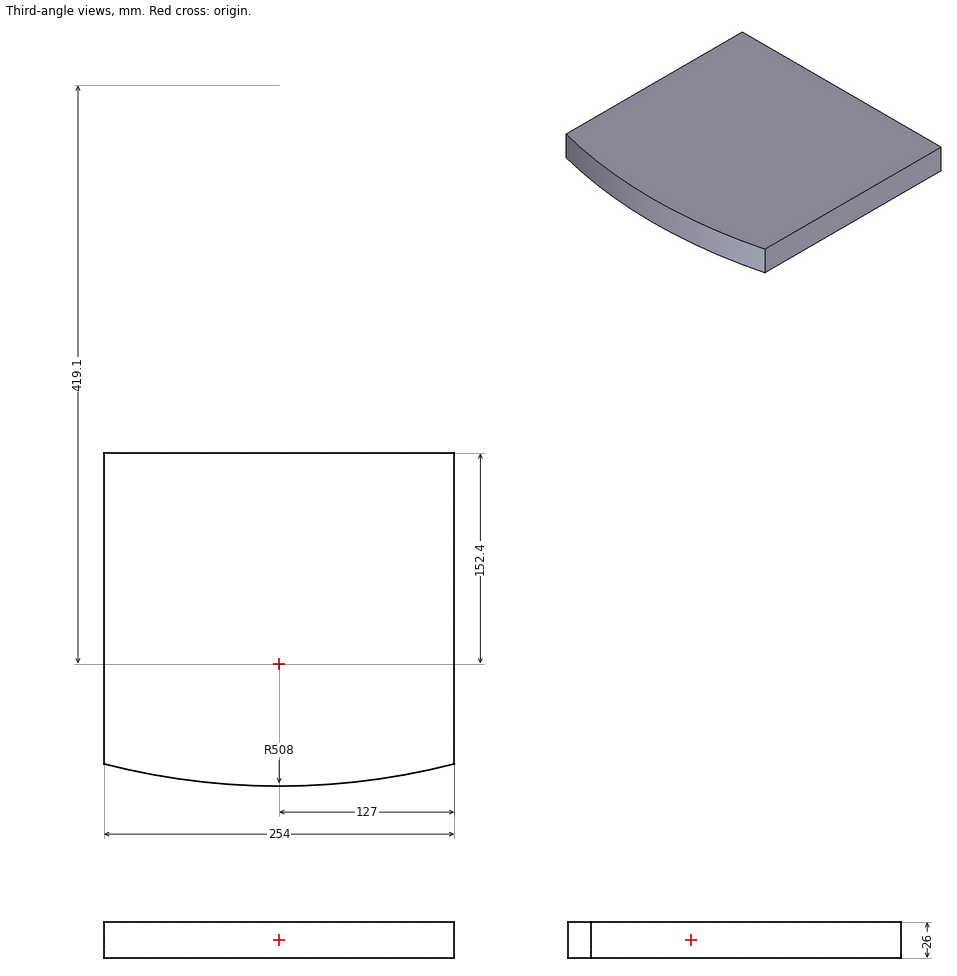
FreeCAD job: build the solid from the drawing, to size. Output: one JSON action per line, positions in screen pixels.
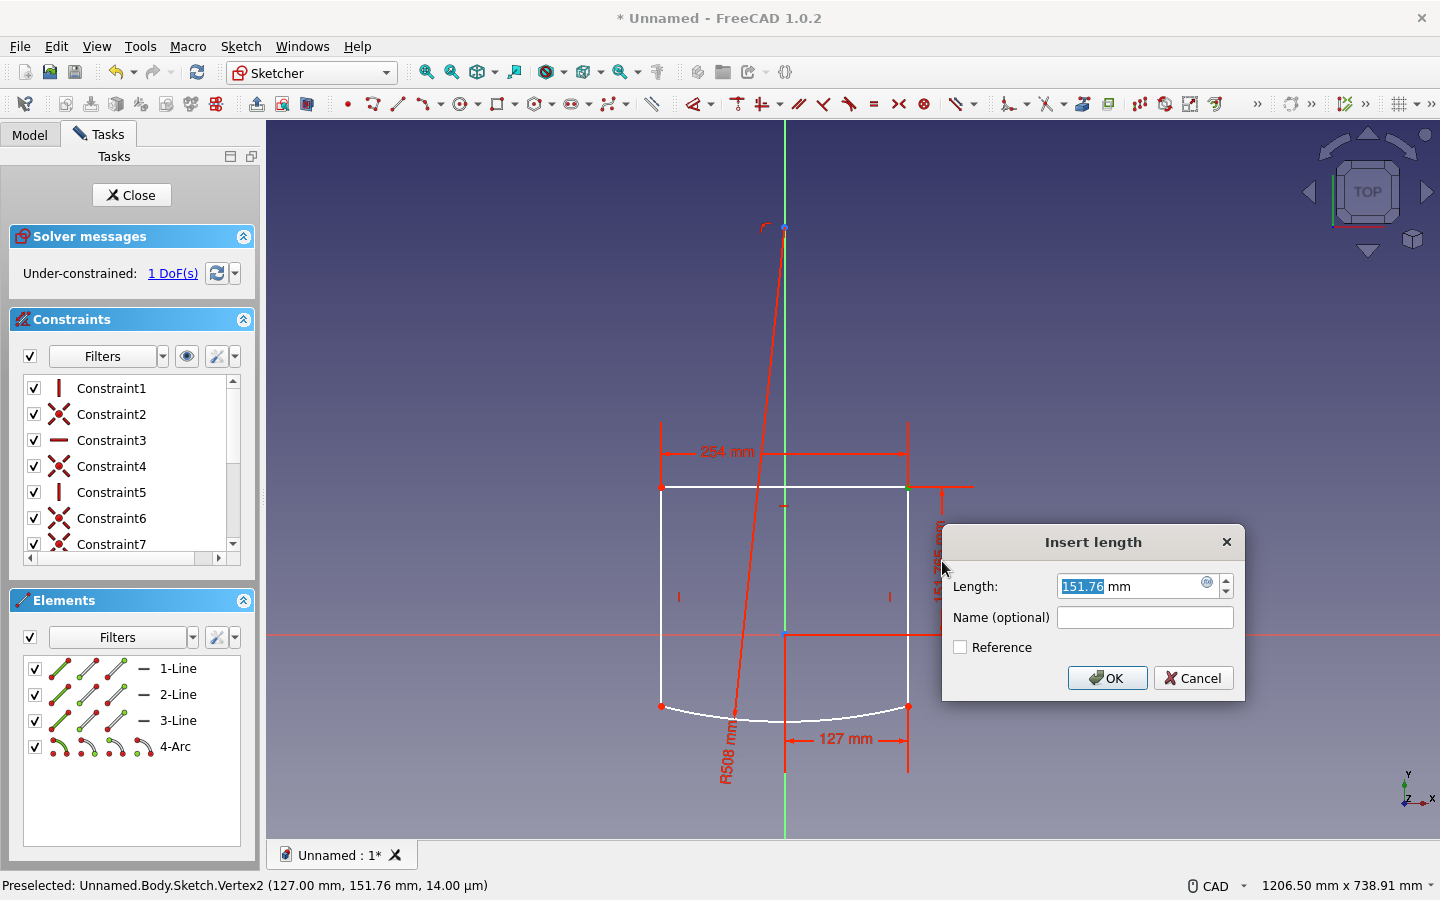
{"action": "type", "text": "152.4"}
{"action": "key", "text": "Return"}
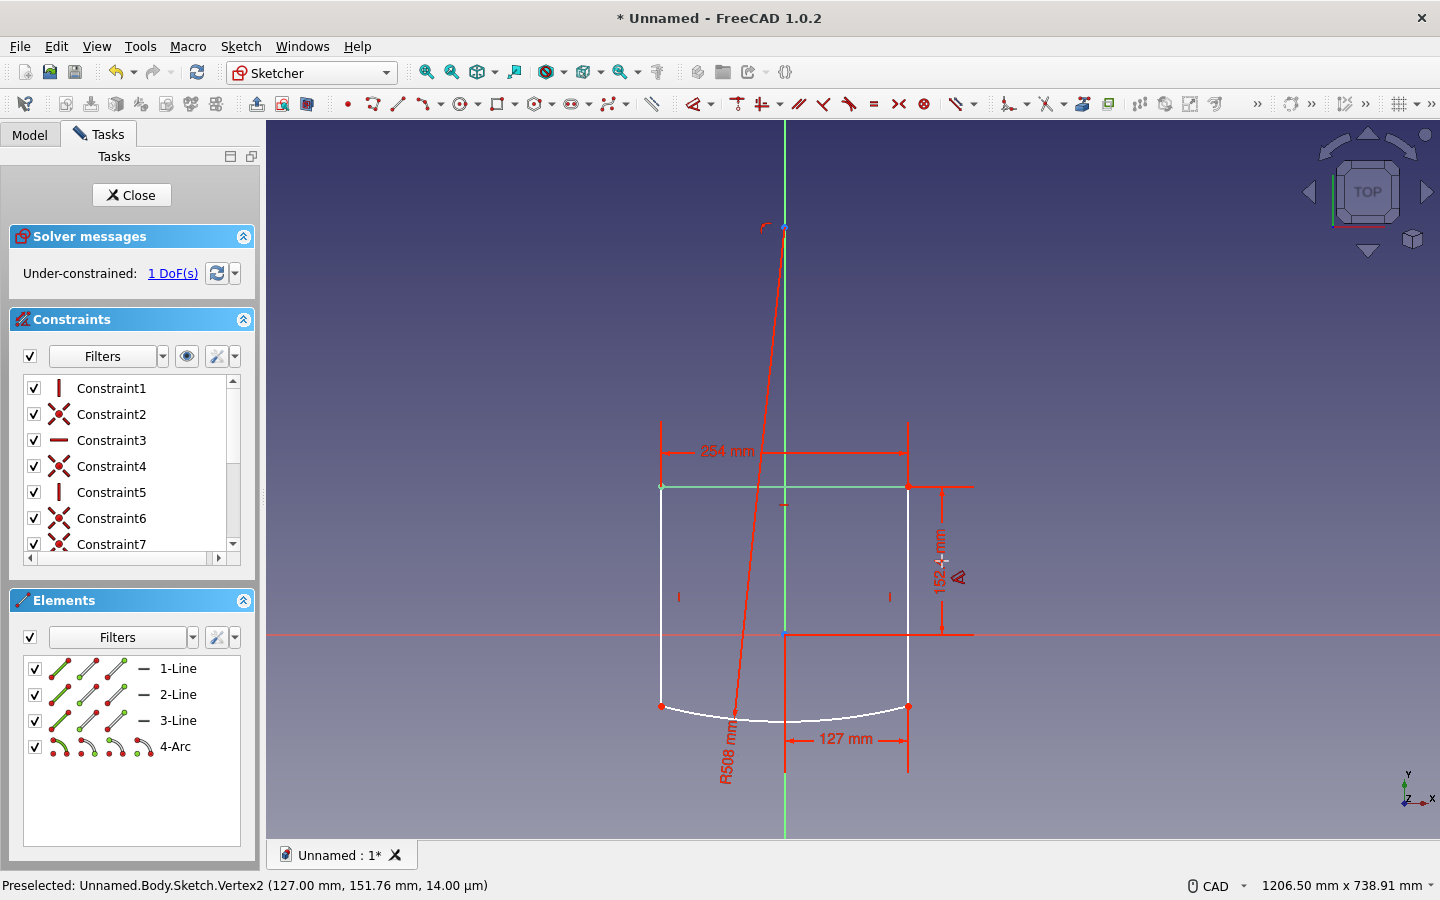
{"action": "left_click", "coordinate": [785, 227]}
{"action": "left_click", "coordinate": [819, 431]}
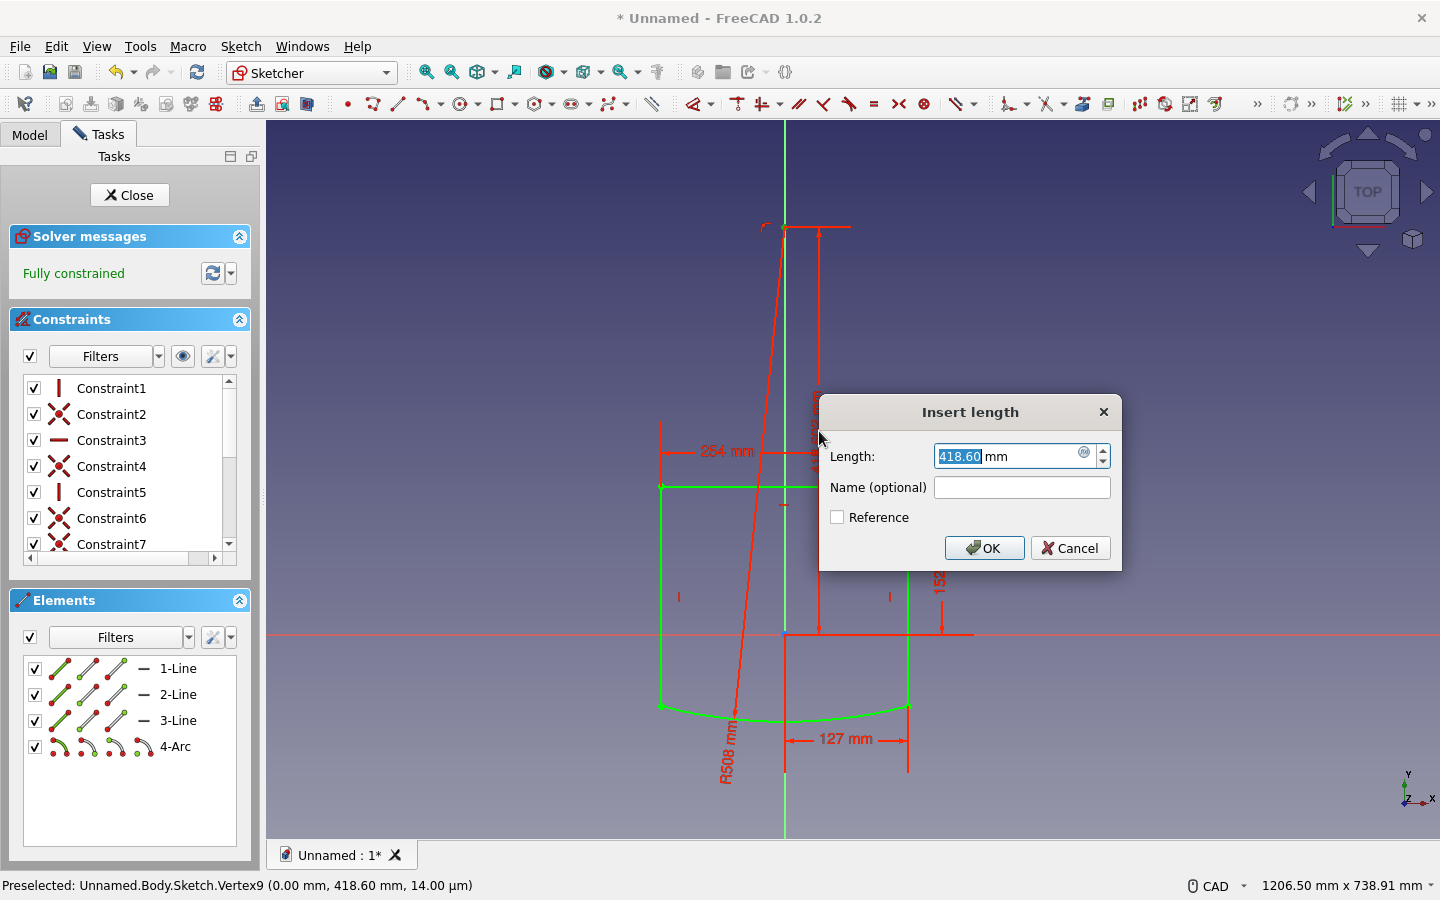
{"action": "type", "text": "419.1"}
{"action": "key", "text": "Return"}
{"action": "key", "text": "Escape"}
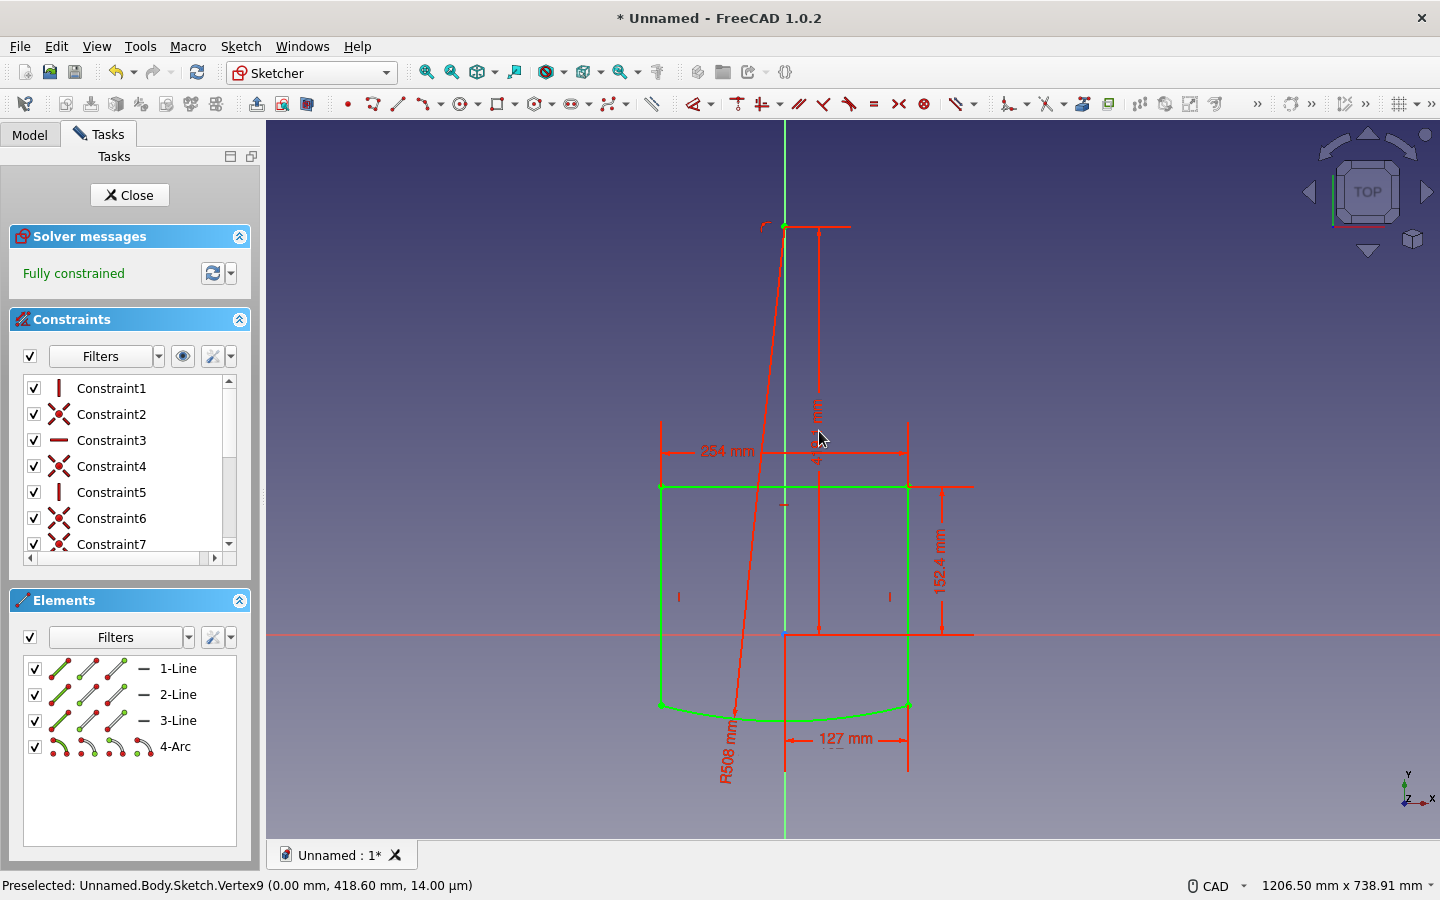
{"action": "left_click", "coordinate": [130, 195]}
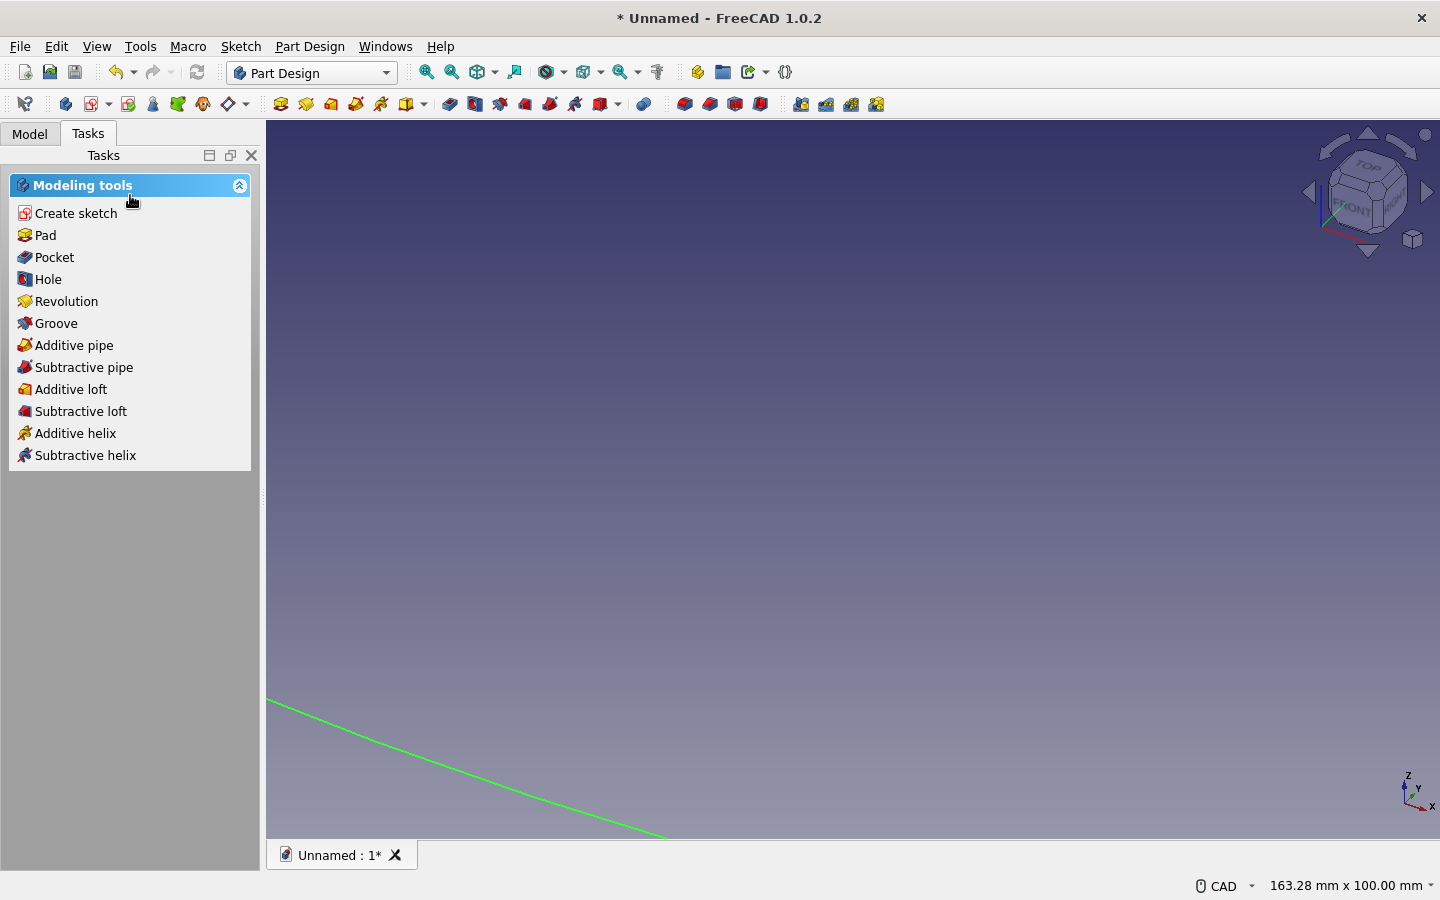
{"action": "left_click", "coordinate": [281, 104]}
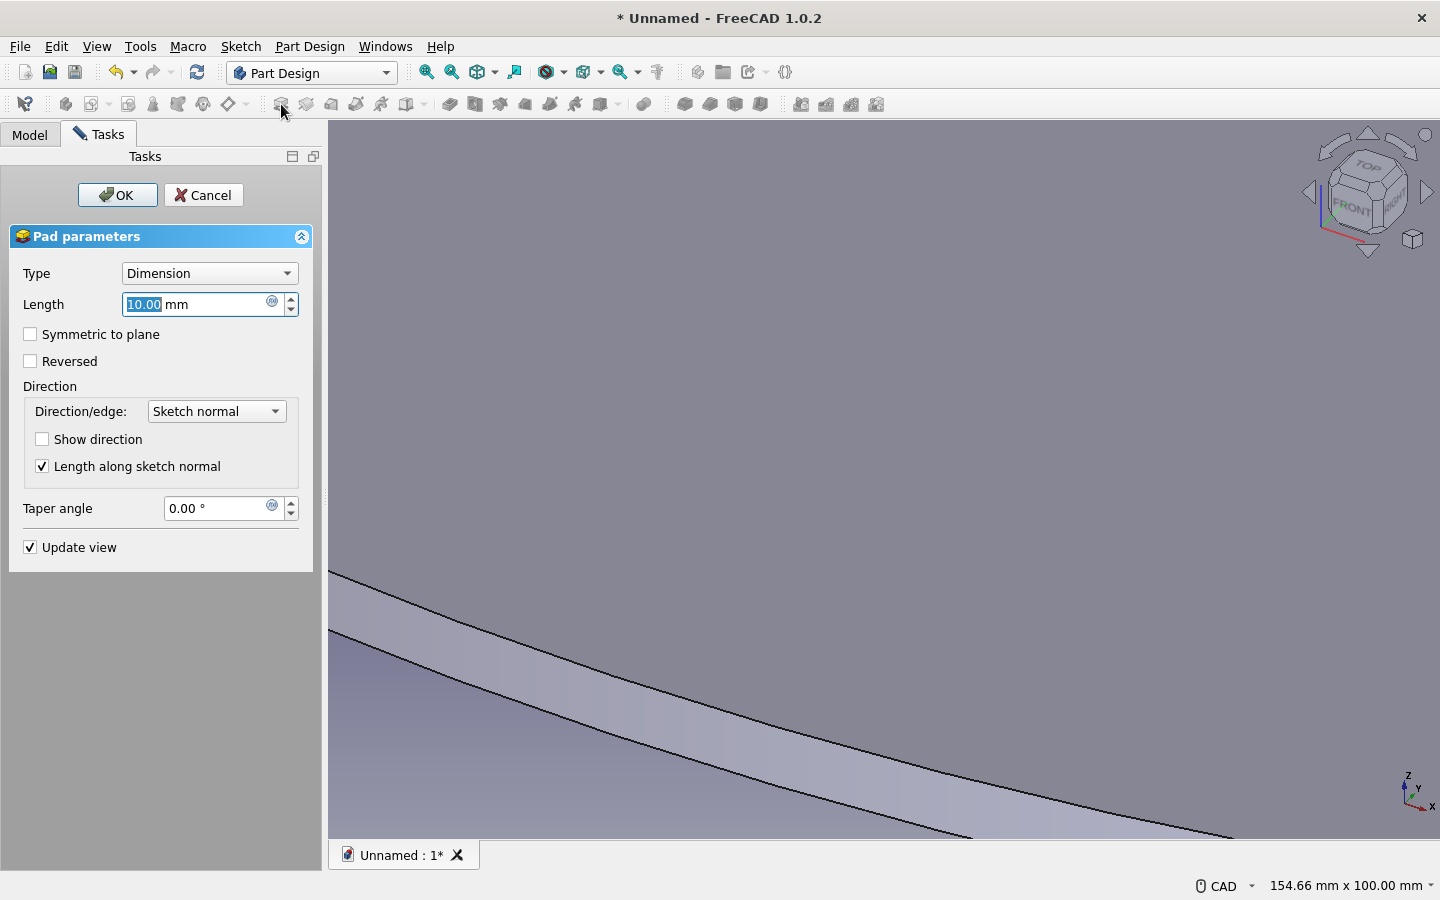
{"action": "type", "text": "26"}
{"action": "key", "text": "Tab"}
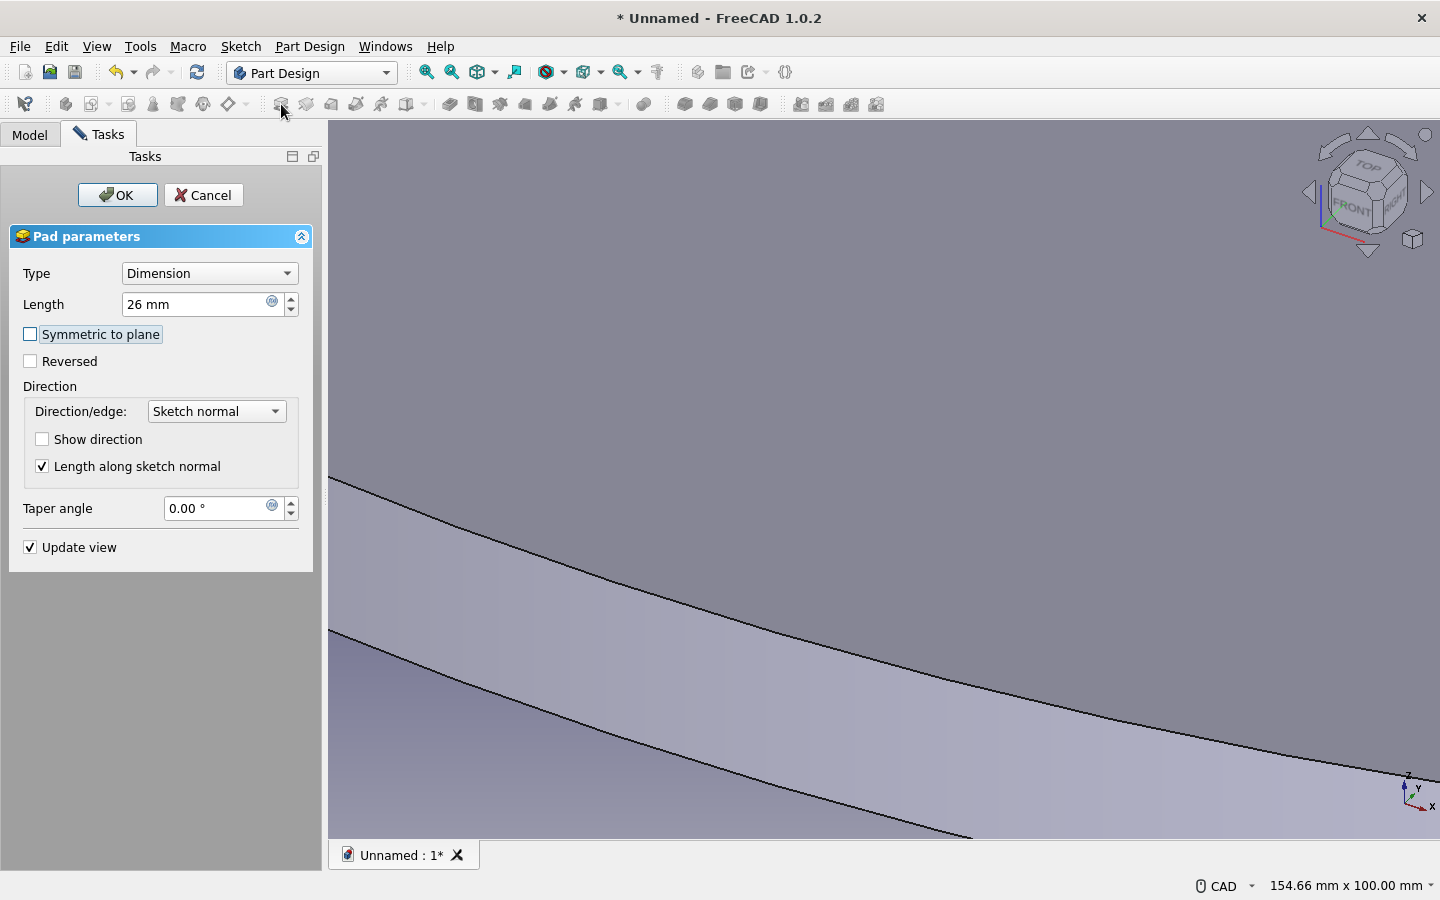
{"action": "left_click", "coordinate": [31, 334]}